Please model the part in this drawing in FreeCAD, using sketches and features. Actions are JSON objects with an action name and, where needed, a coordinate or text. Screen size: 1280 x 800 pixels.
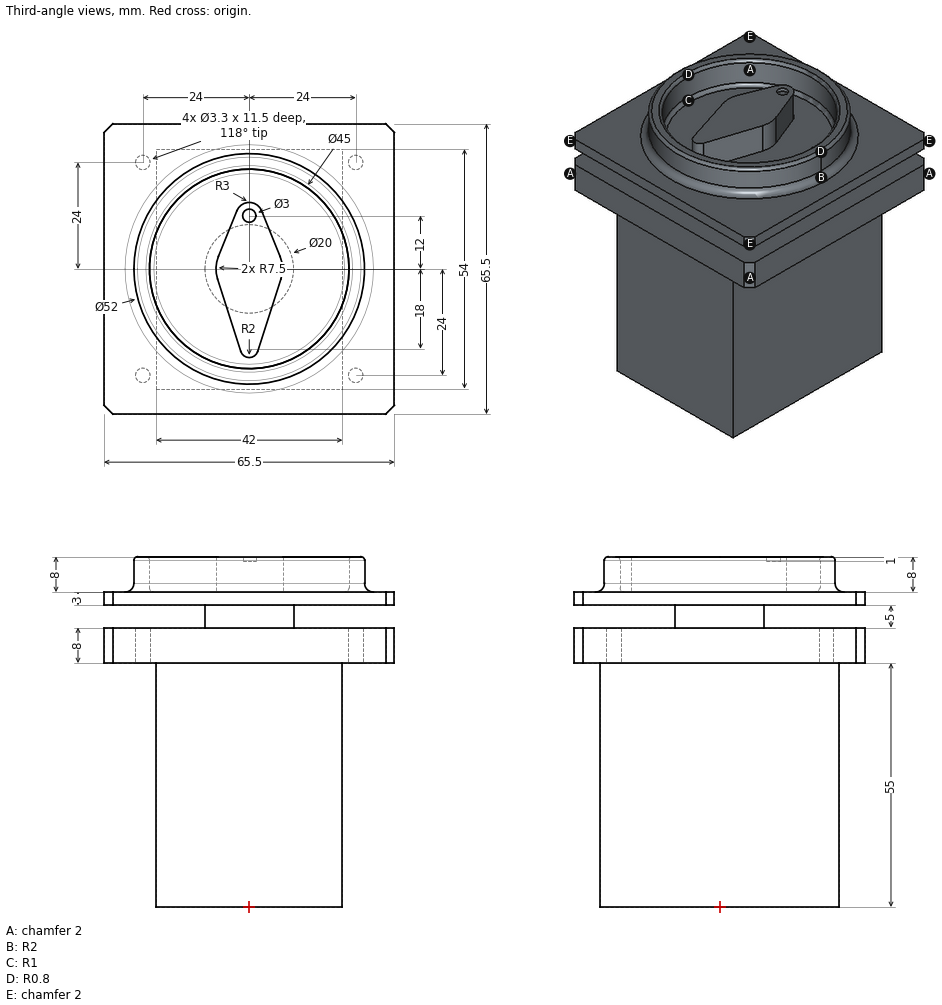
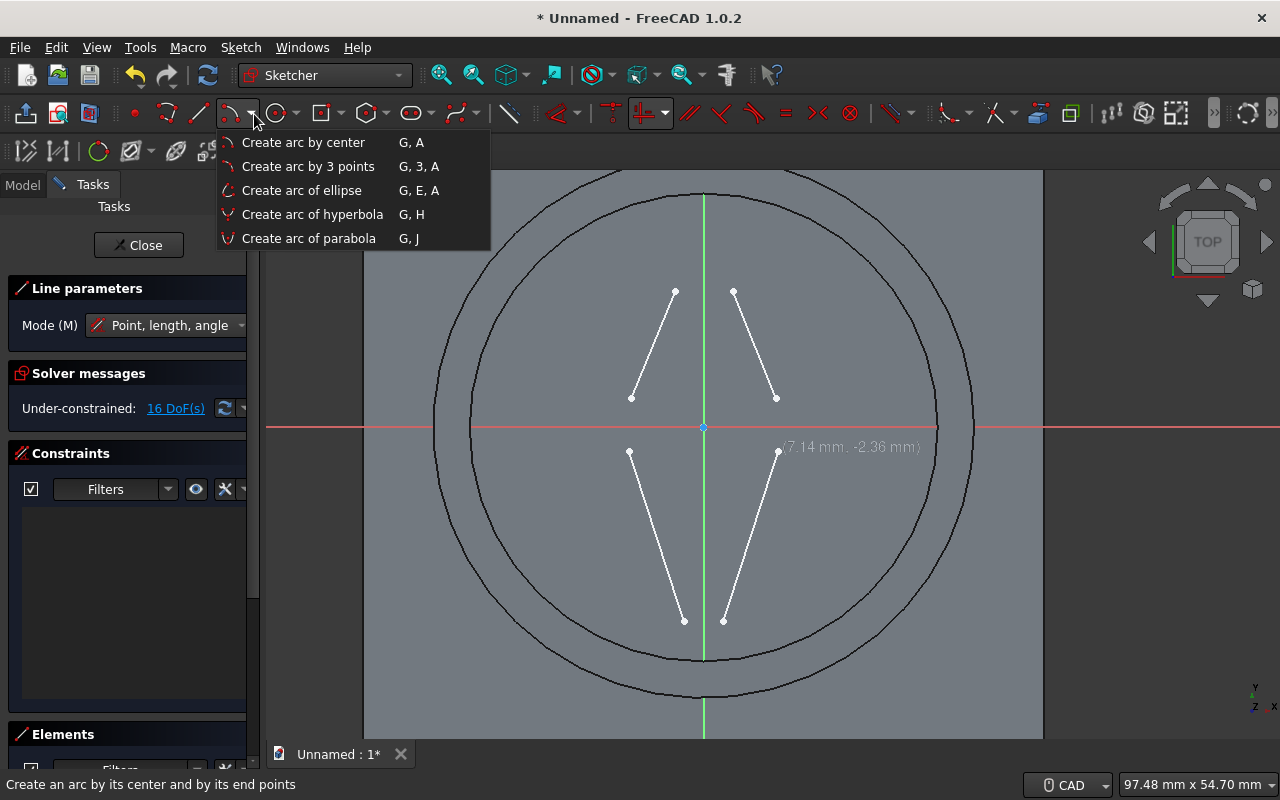
{"action": "left_click", "coordinate": [354, 166]}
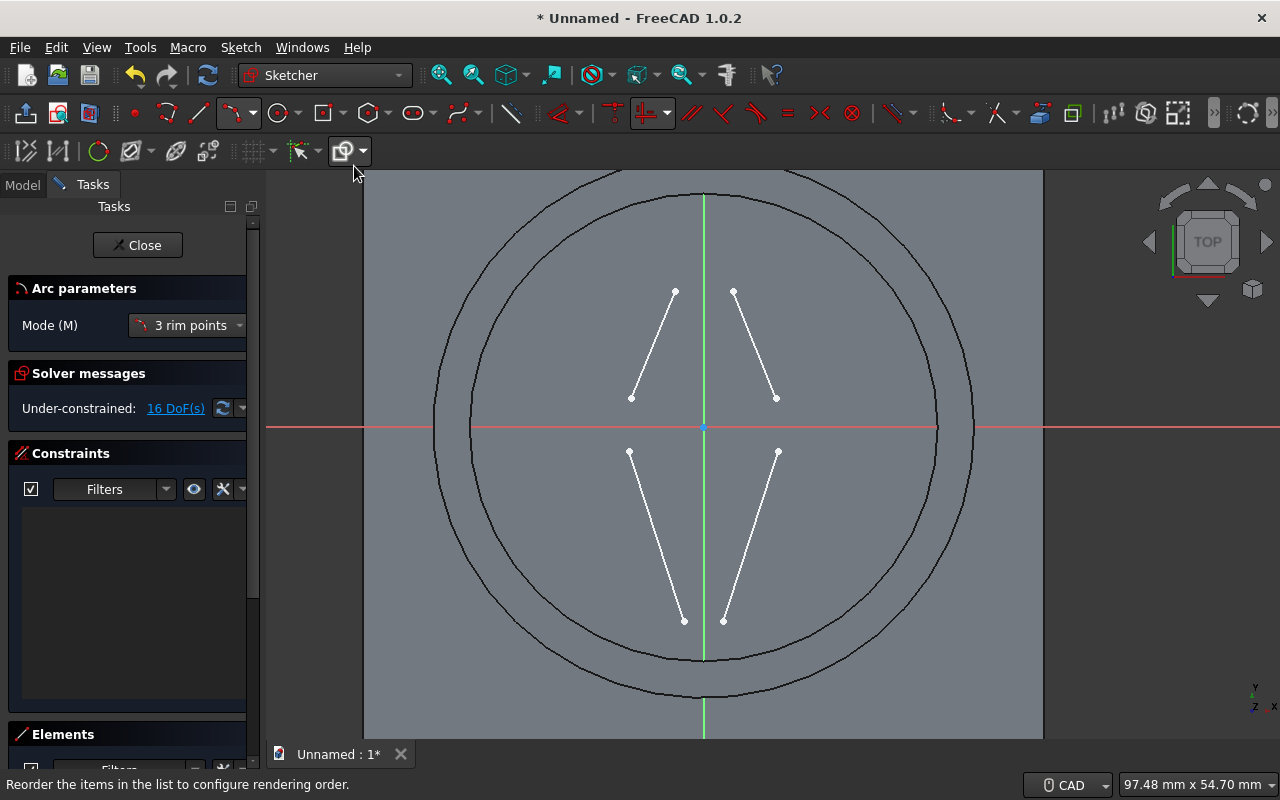
{"action": "left_click", "coordinate": [733, 292]}
{"action": "left_click", "coordinate": [675, 292]}
{"action": "left_click", "coordinate": [718, 275]}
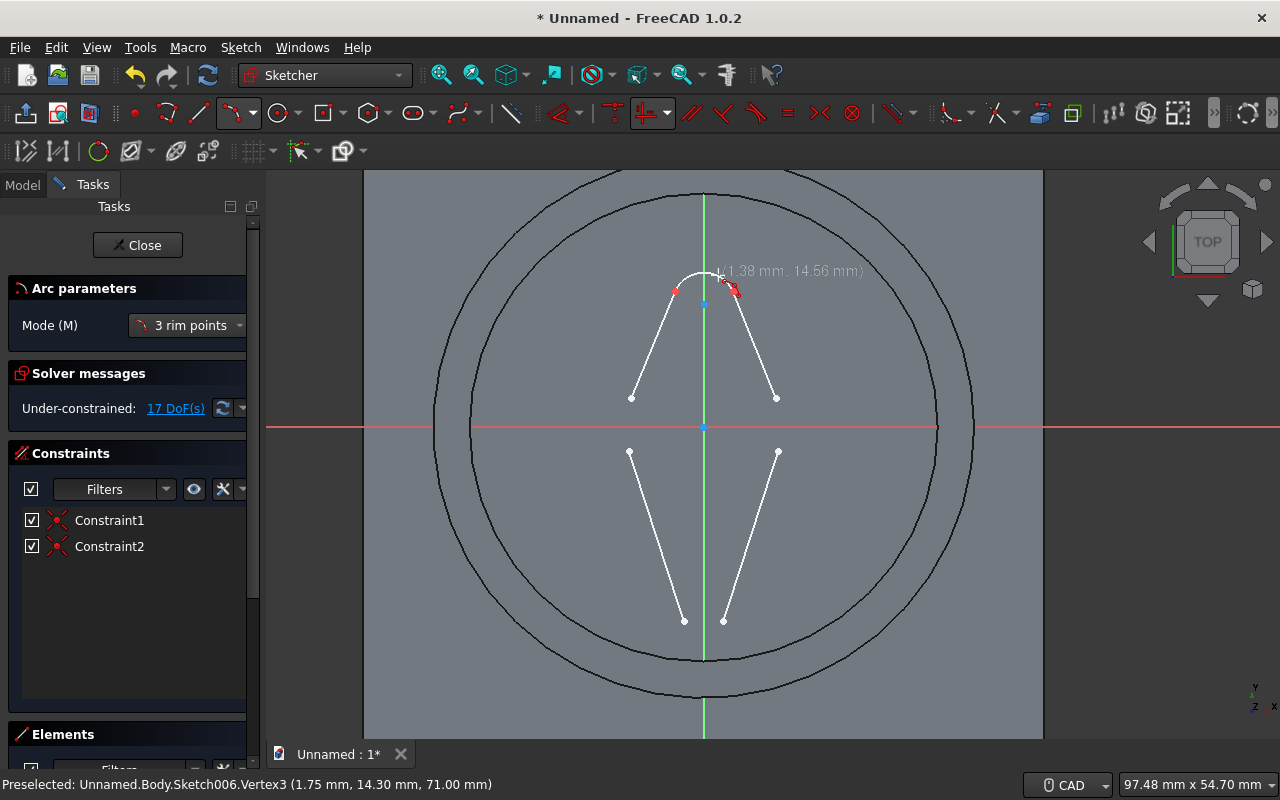
{"action": "left_click", "coordinate": [631, 399]}
{"action": "left_click", "coordinate": [629, 452]}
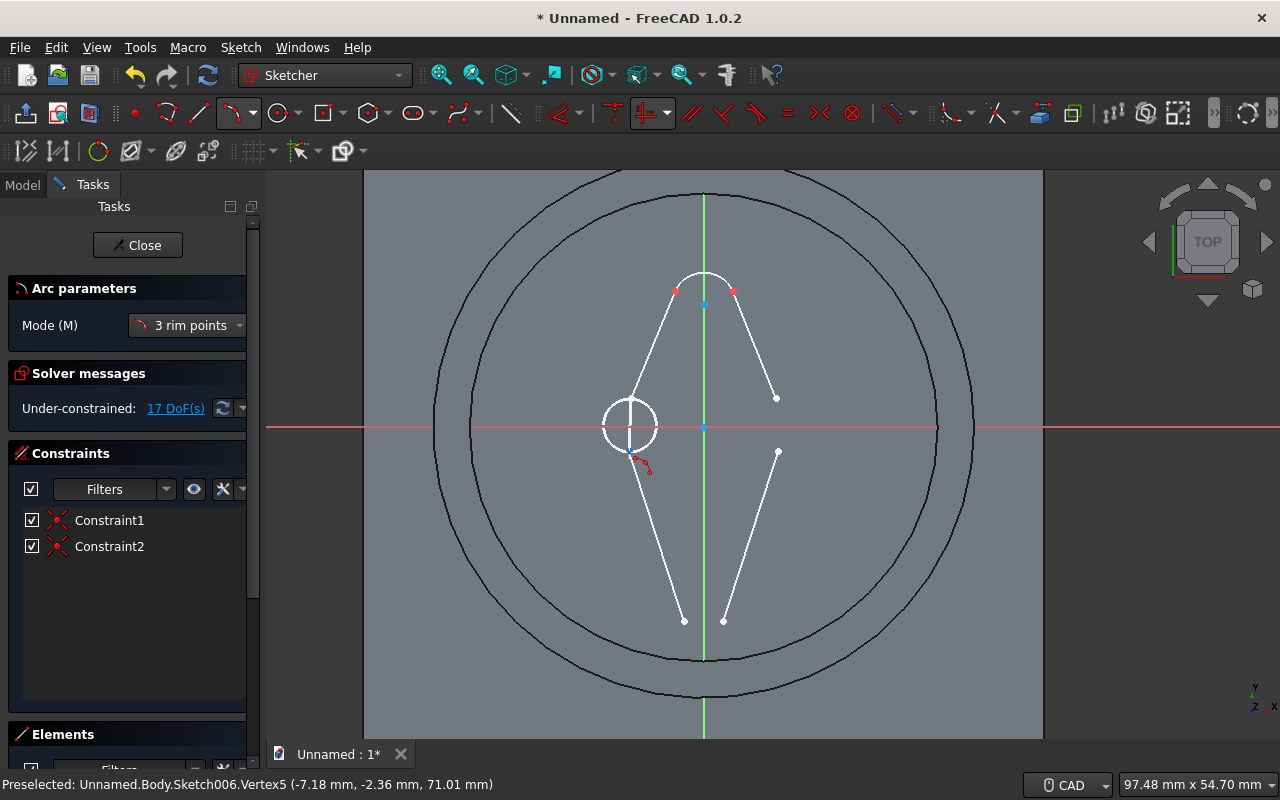
{"action": "scroll", "coordinate": [626, 419], "scroll_direction": "up", "scroll_amount": 7}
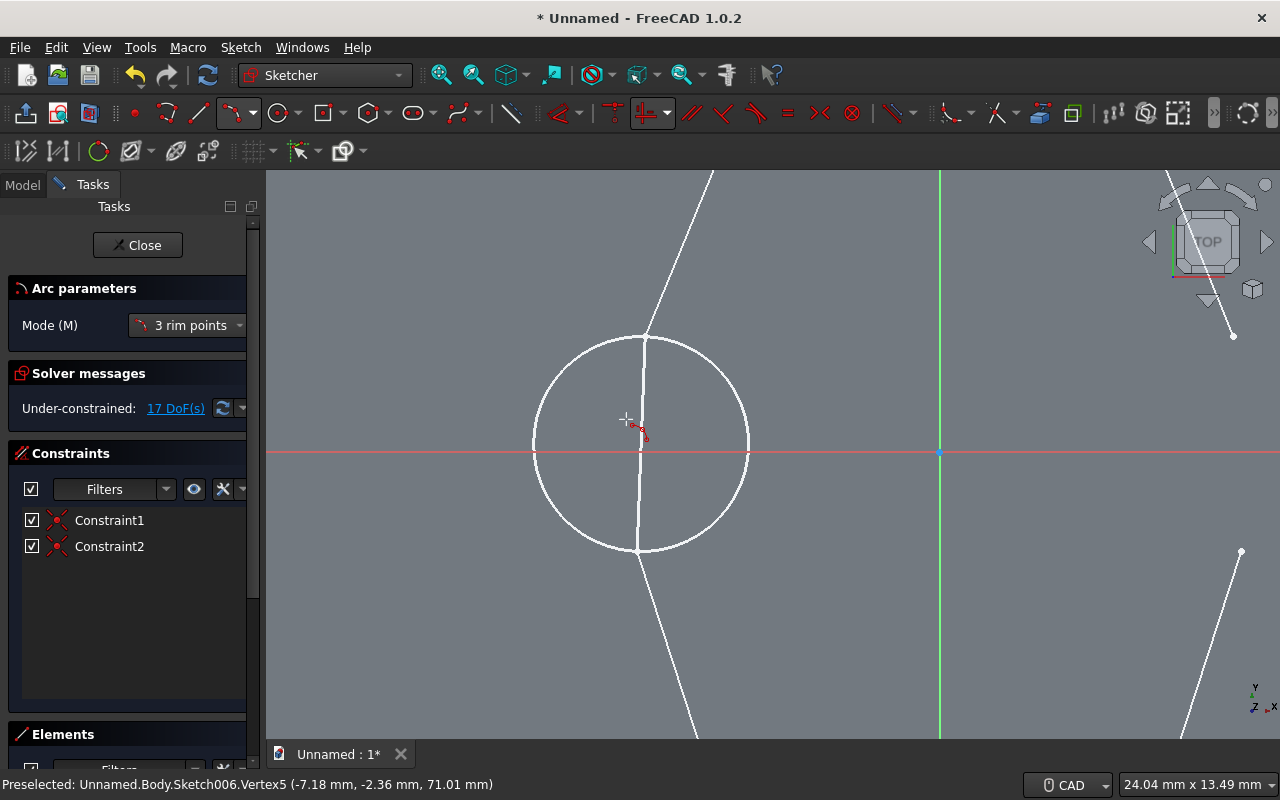
{"action": "left_click", "coordinate": [625, 418]}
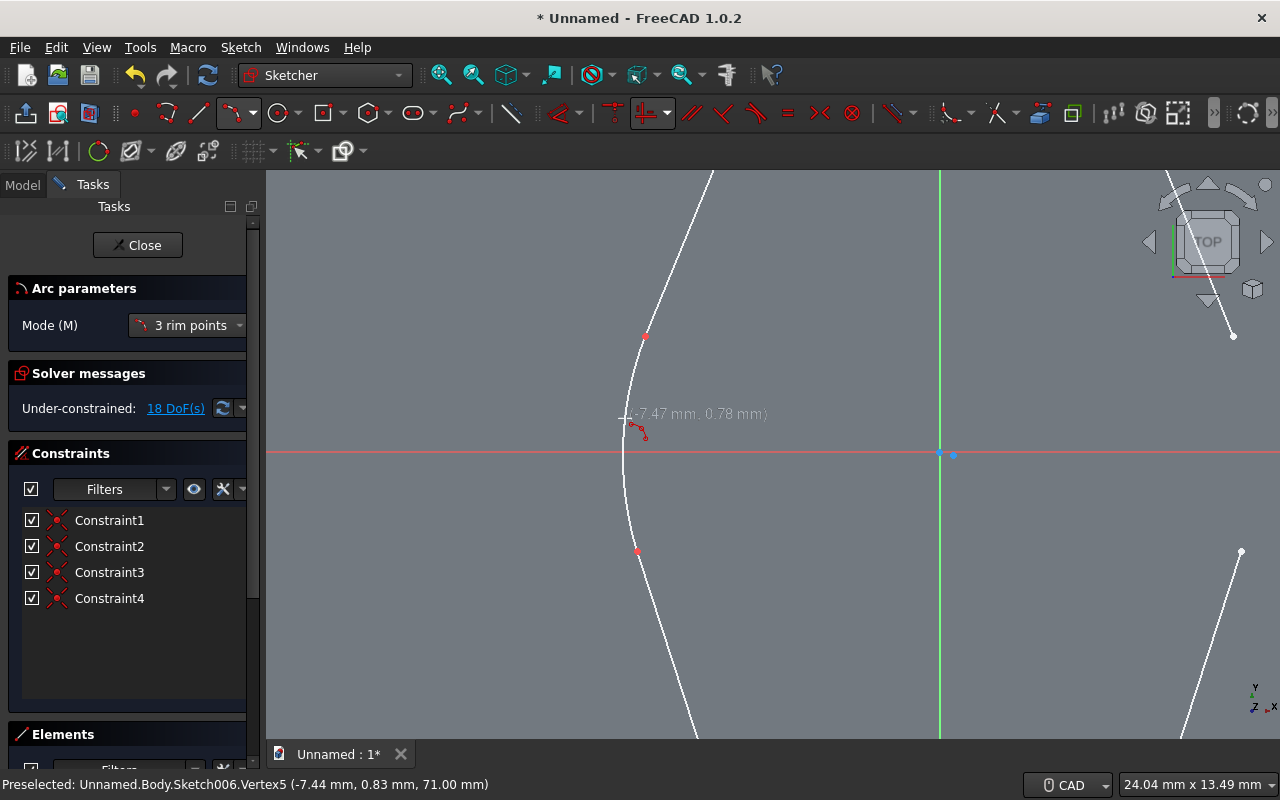
{"action": "scroll", "coordinate": [627, 421], "scroll_direction": "down", "scroll_amount": 7}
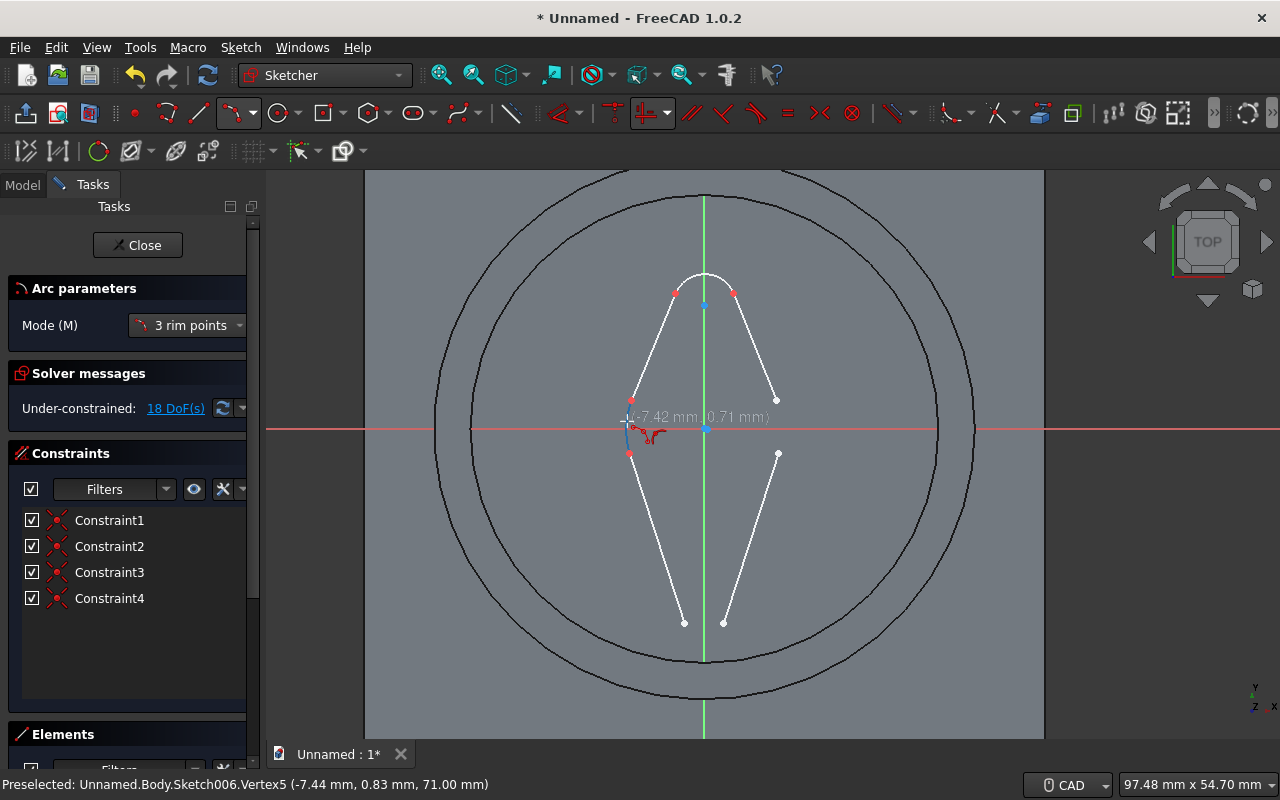
{"action": "left_click", "coordinate": [685, 624]}
{"action": "left_click", "coordinate": [724, 624]}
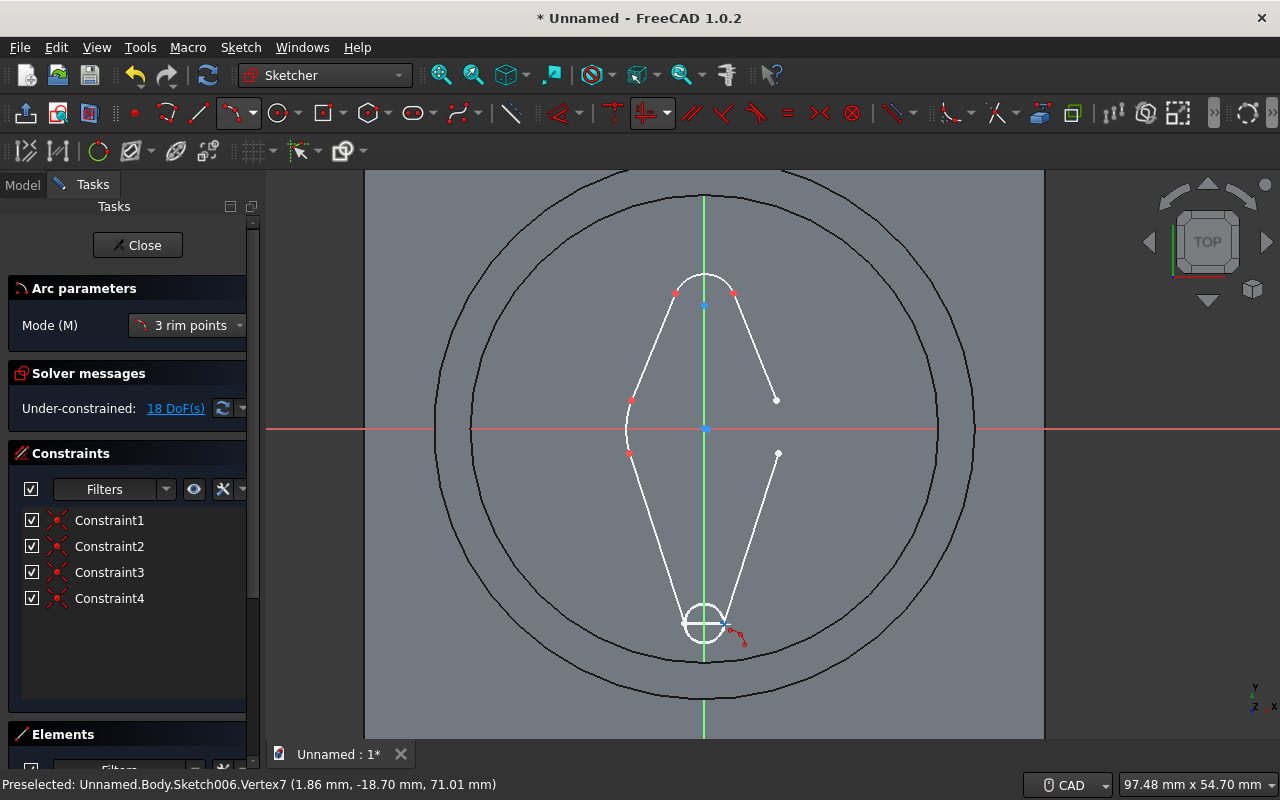
{"action": "scroll", "coordinate": [694, 634], "scroll_direction": "up", "scroll_amount": 3}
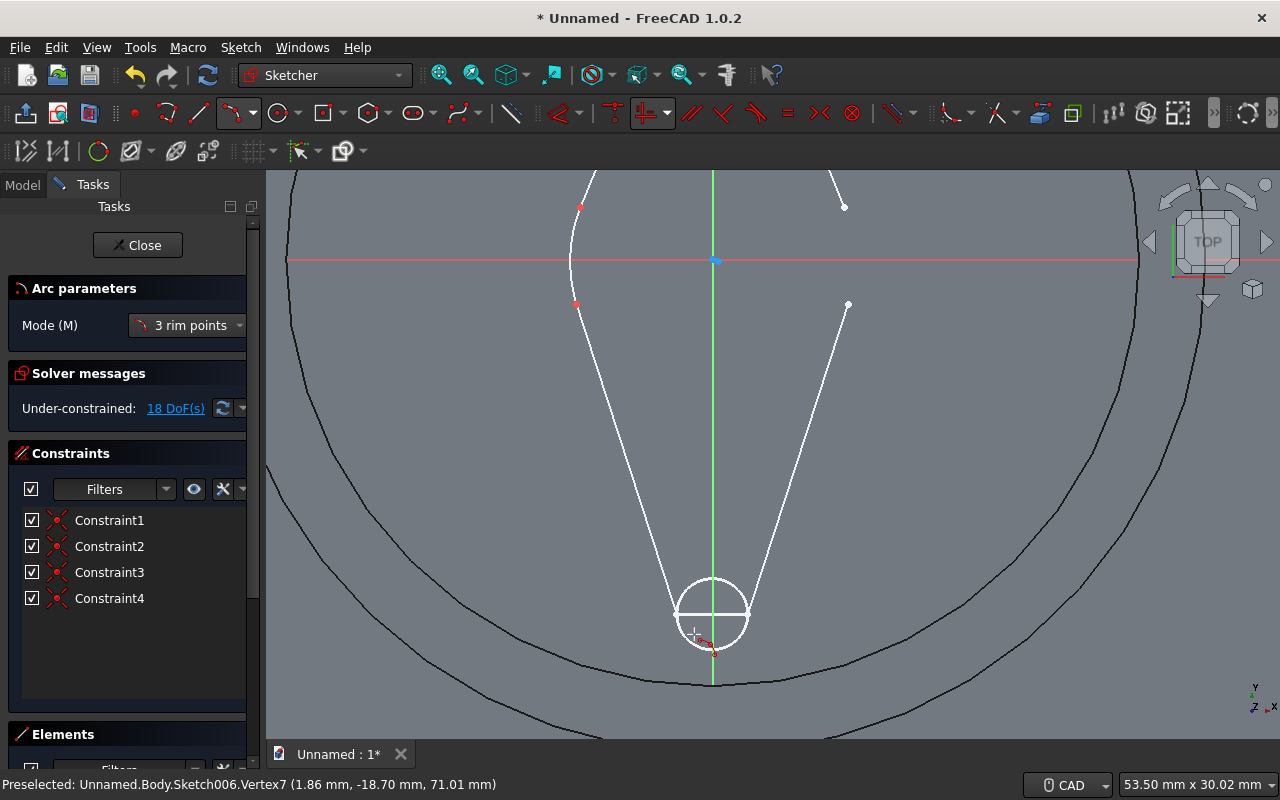
{"action": "left_click", "coordinate": [694, 634]}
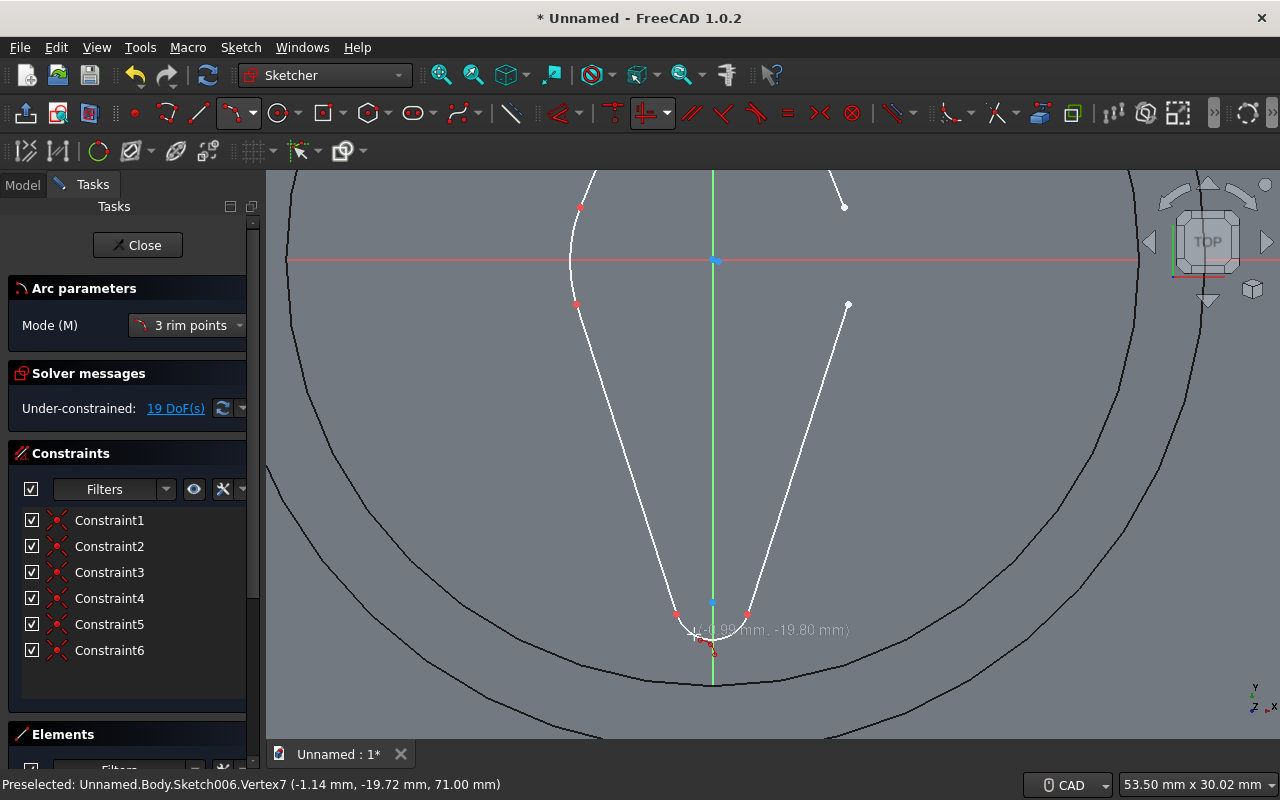
{"action": "left_click", "coordinate": [848, 304]}
{"action": "left_click", "coordinate": [844, 208]}